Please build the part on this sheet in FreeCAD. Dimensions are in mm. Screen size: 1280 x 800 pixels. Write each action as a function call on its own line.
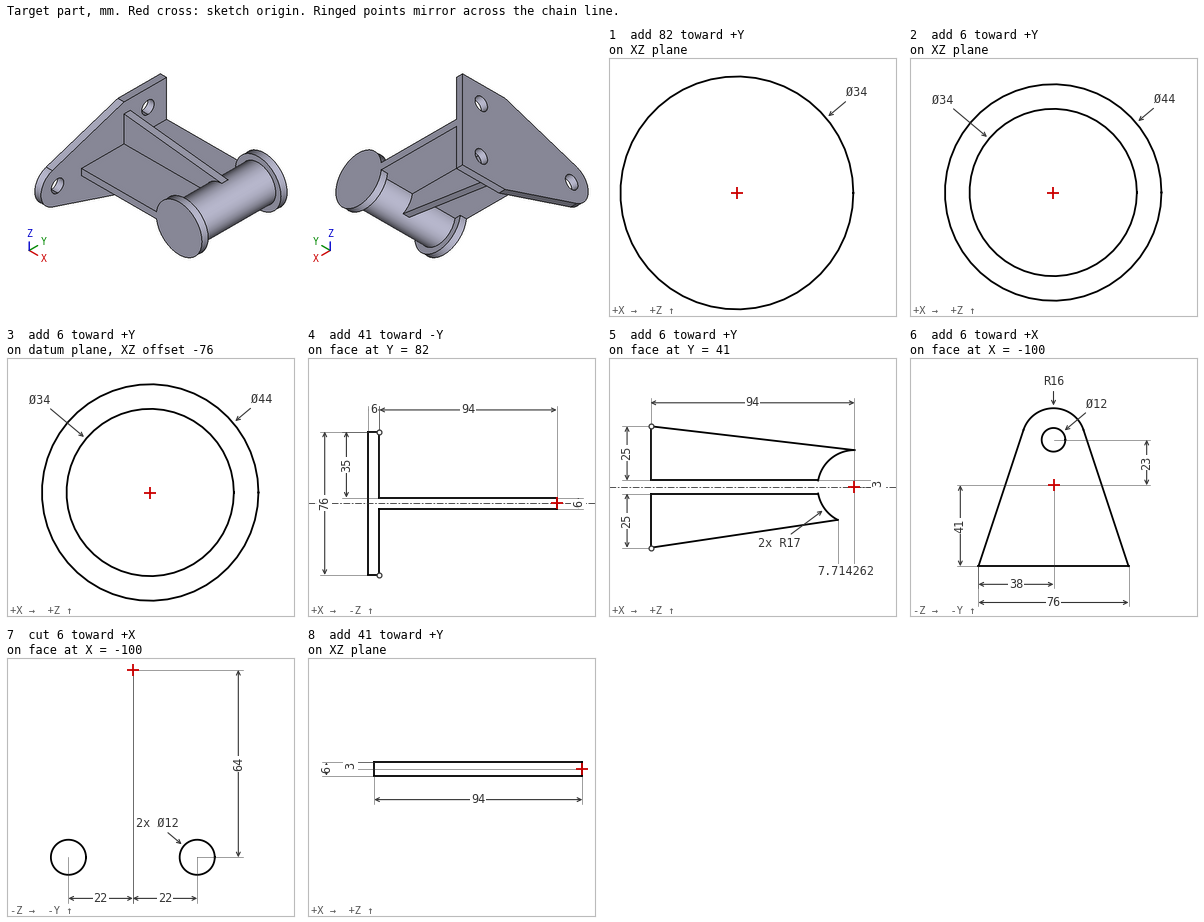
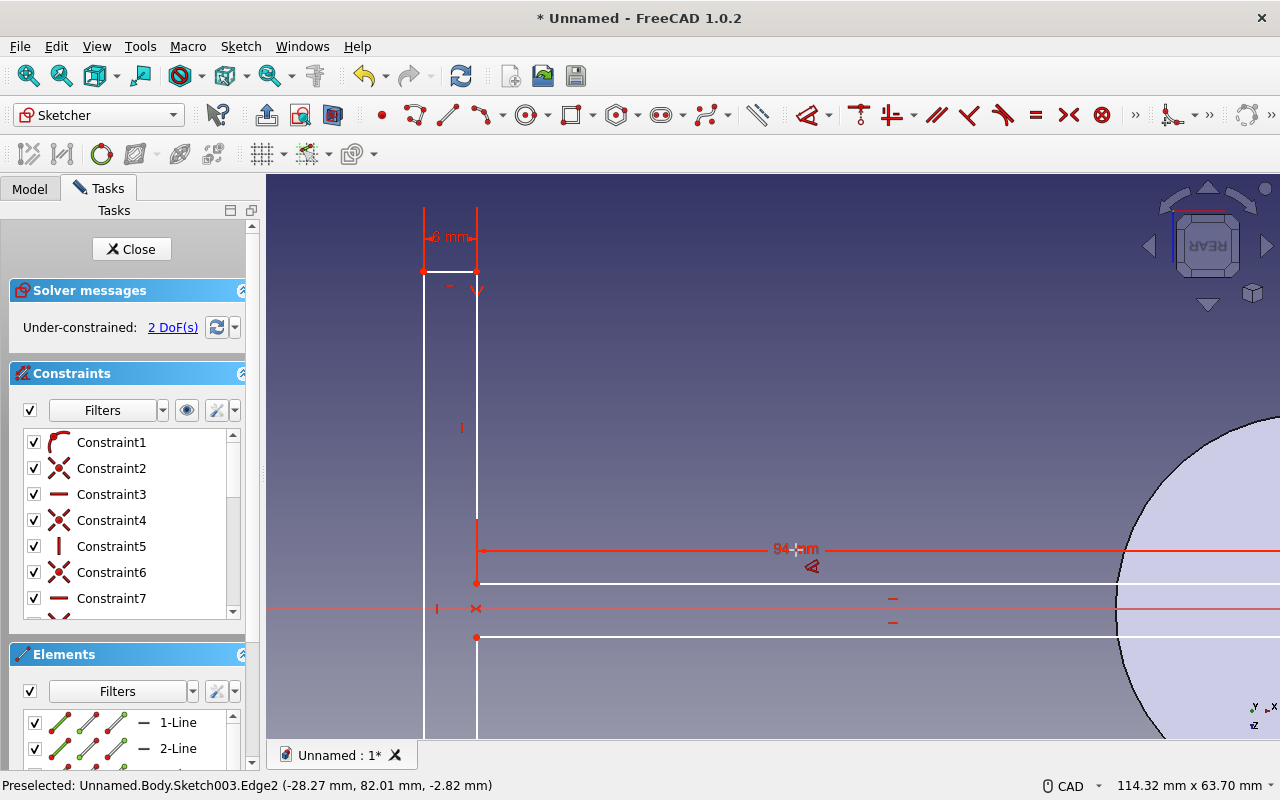
click(477, 490)
click(443, 428)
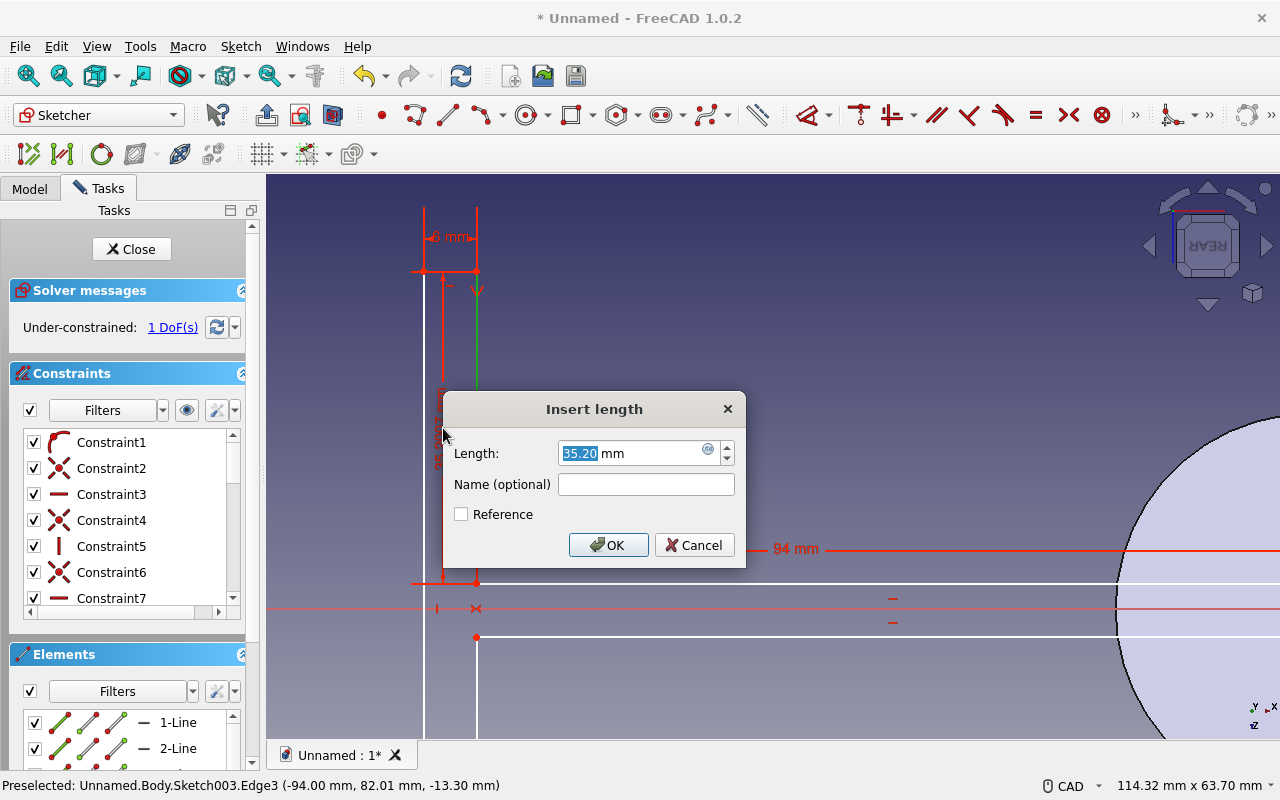
text(35)
key(Return)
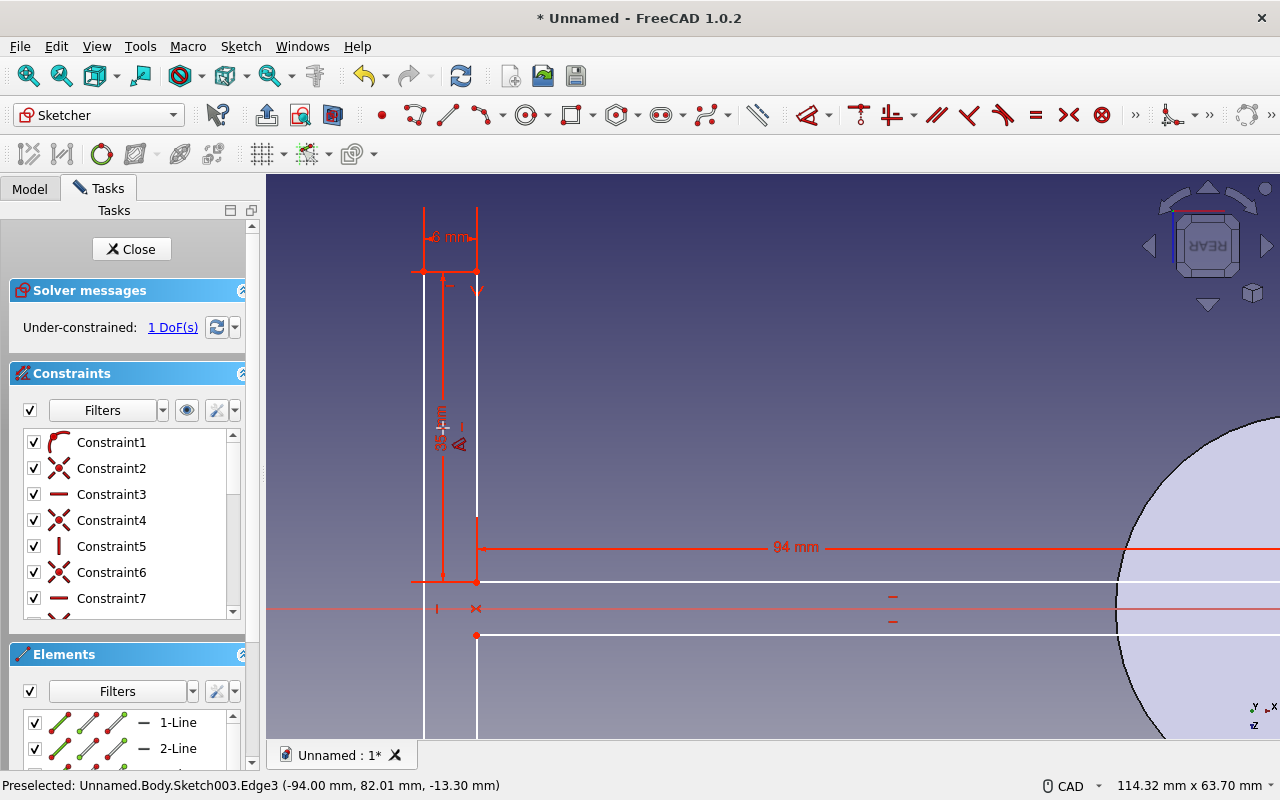
click(424, 474)
click(390, 491)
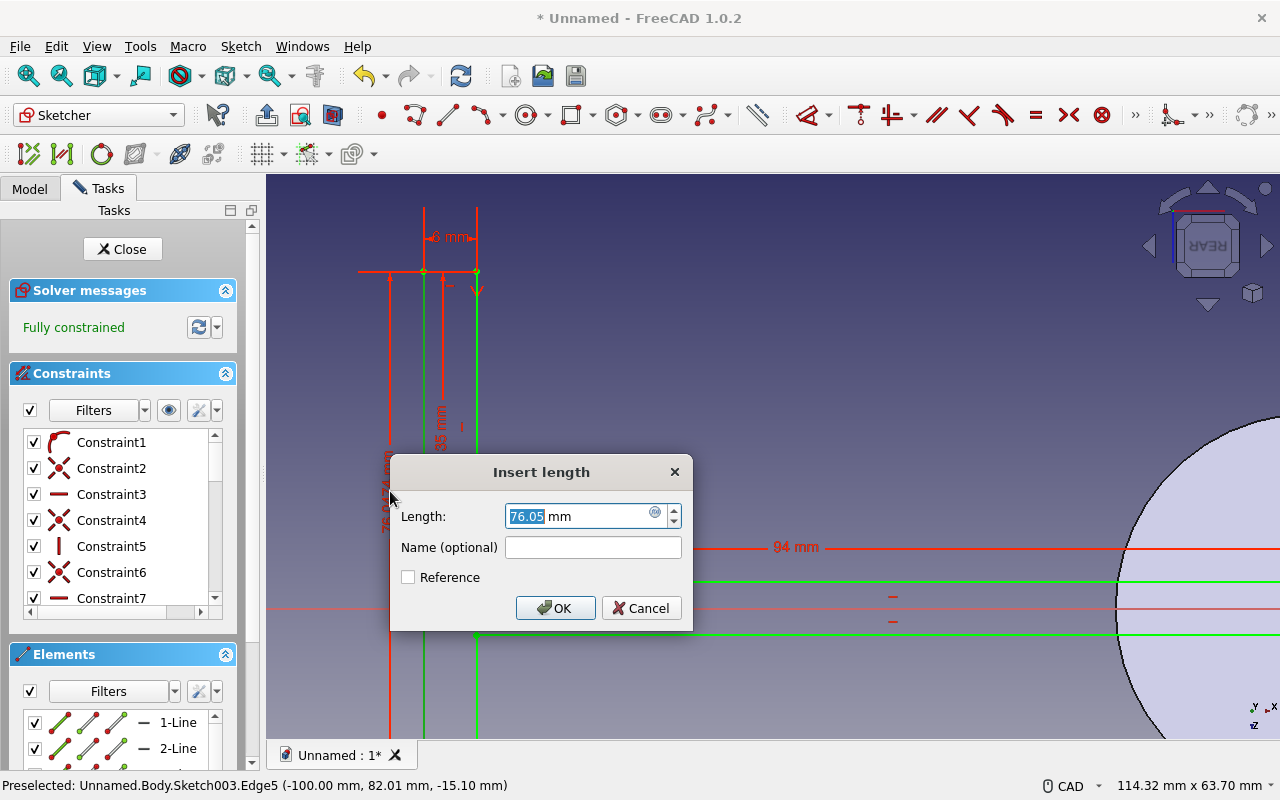
text(76)
key(Return)
key(Escape)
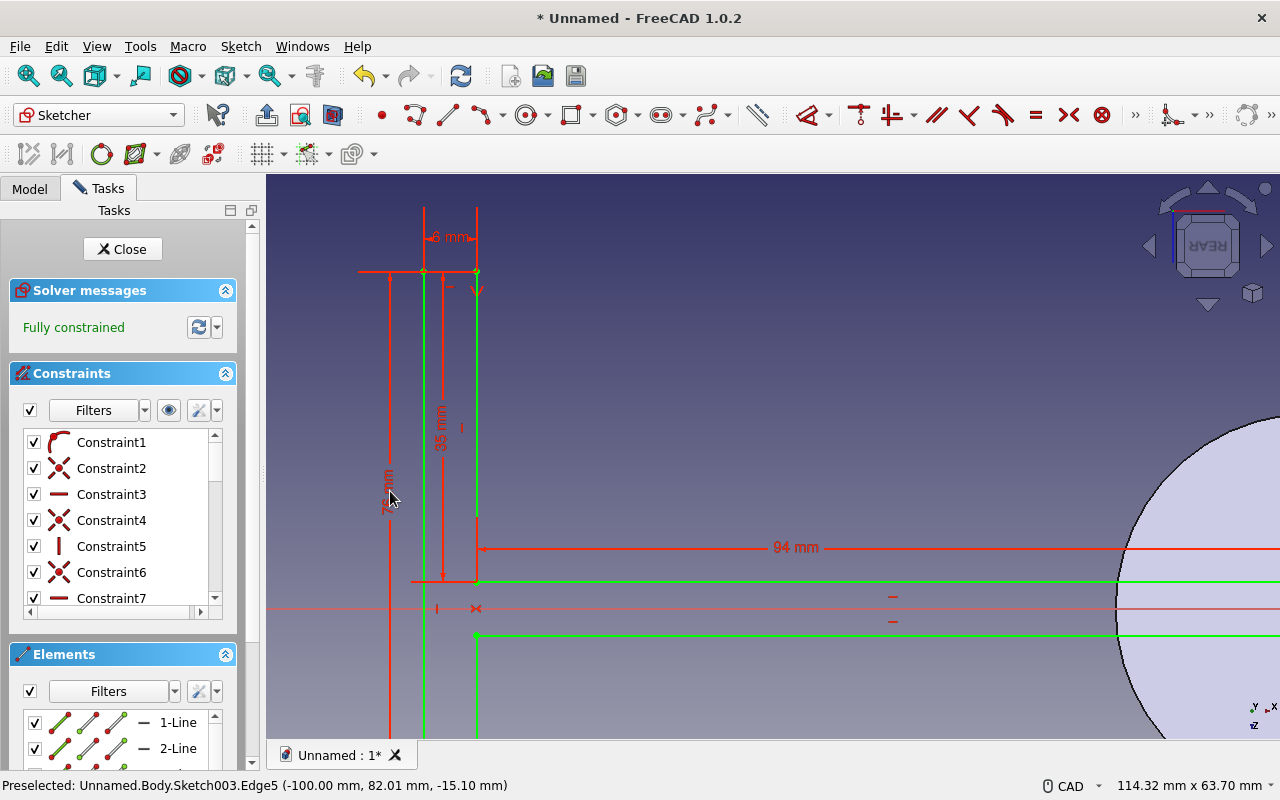
click(123, 249)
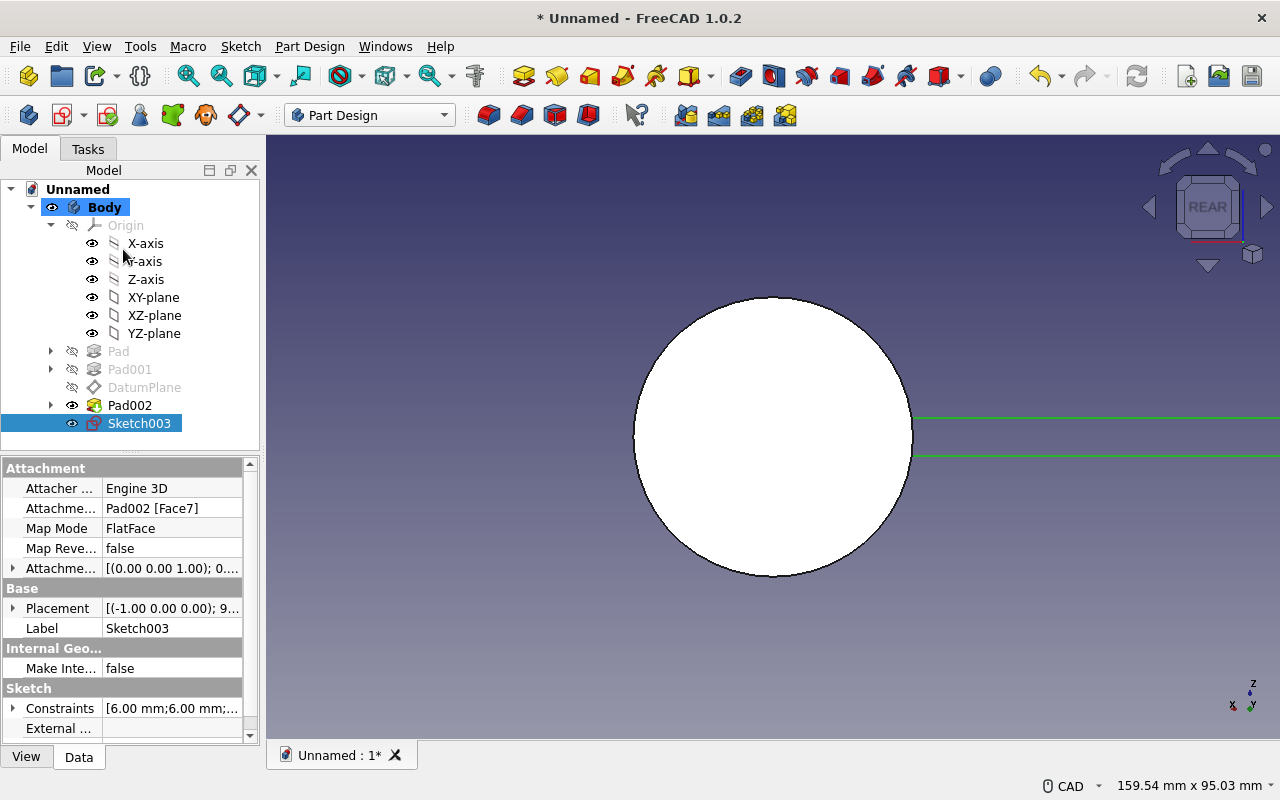
click(524, 76)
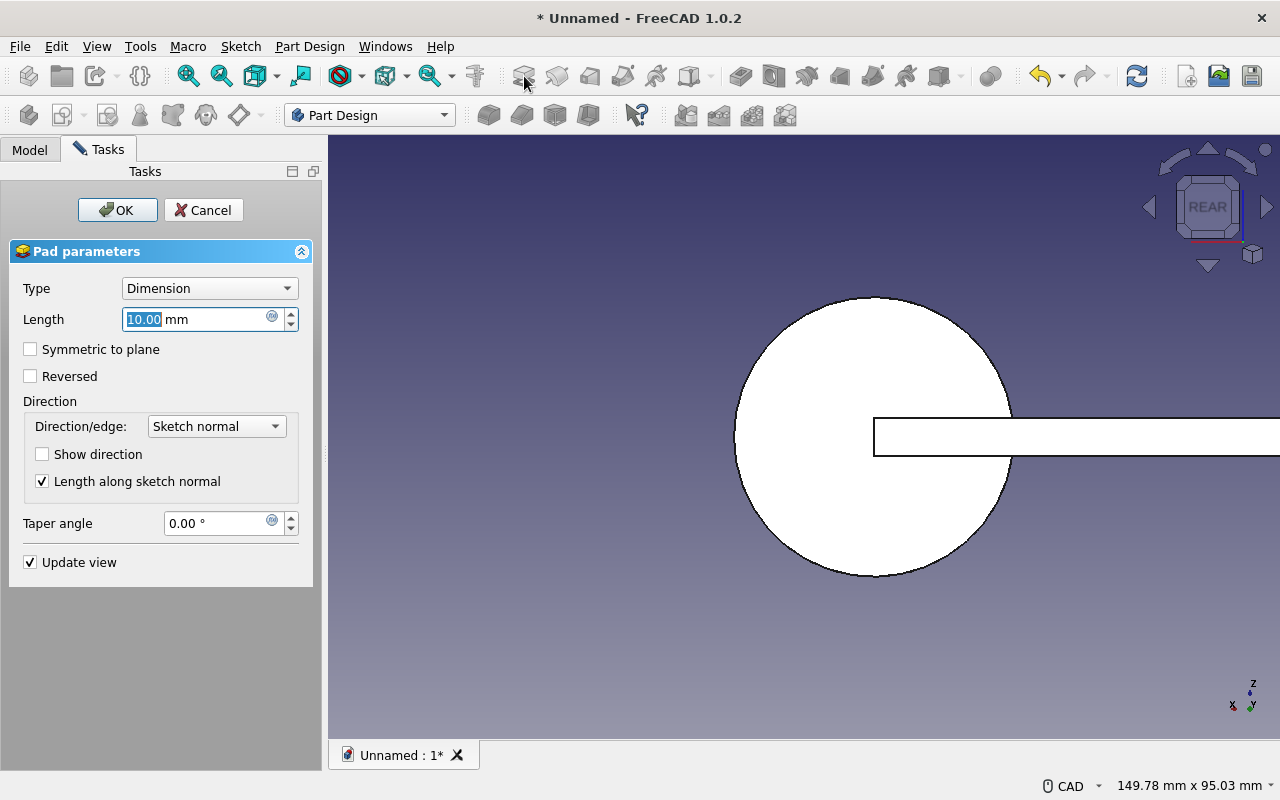
text(41)
key(Tab)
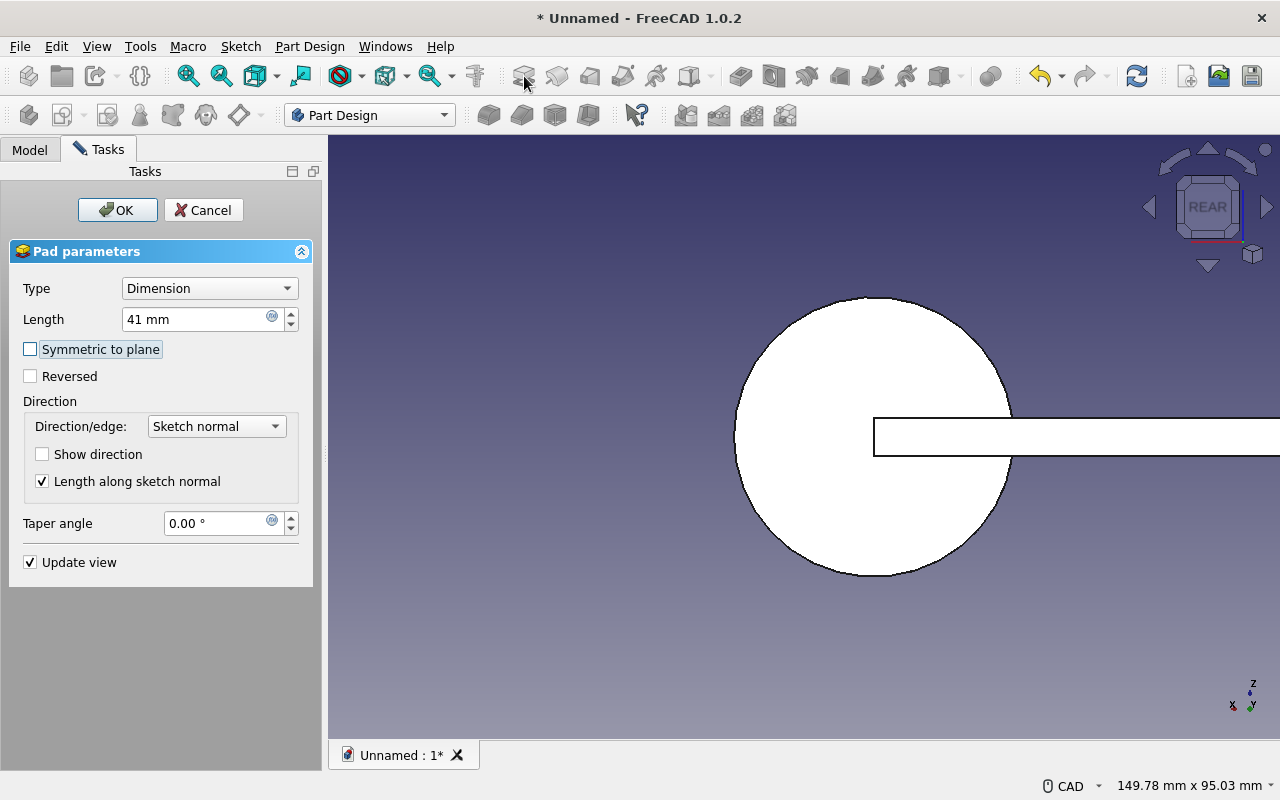
click(31, 376)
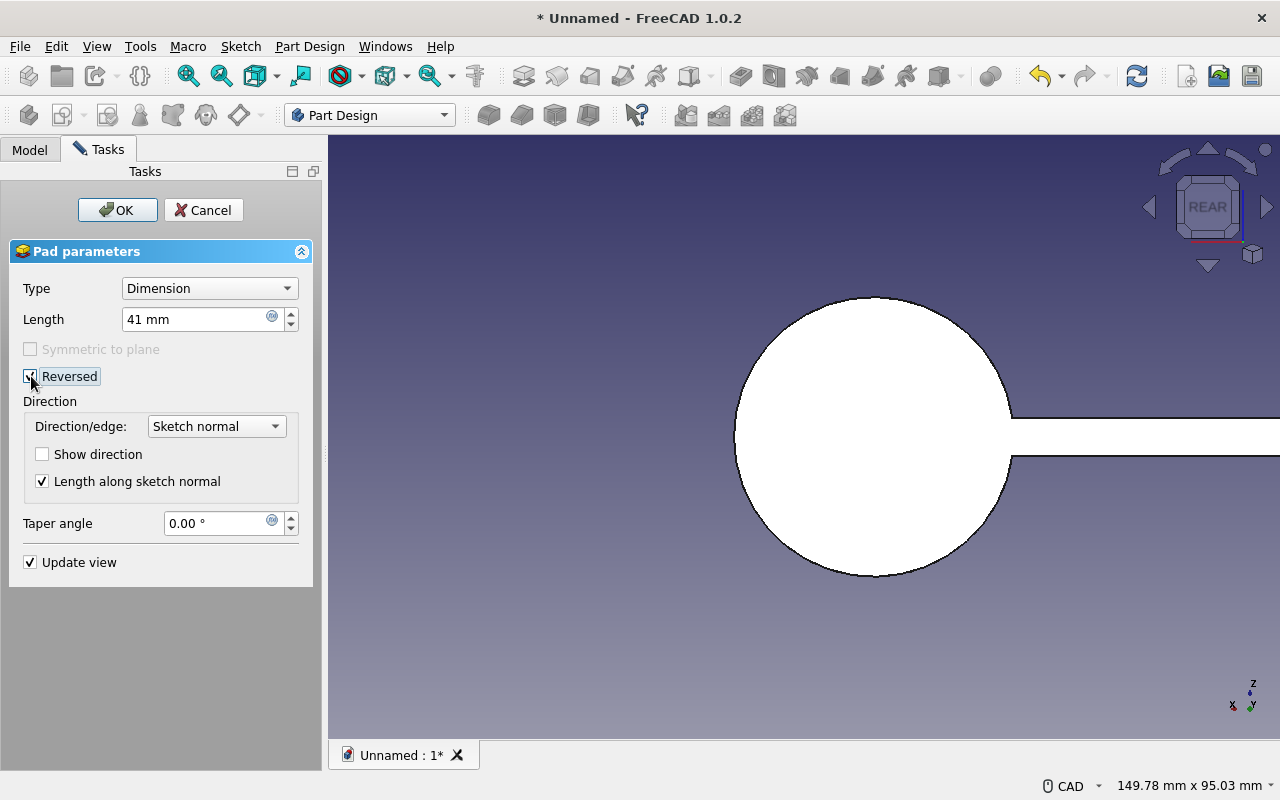
click(118, 210)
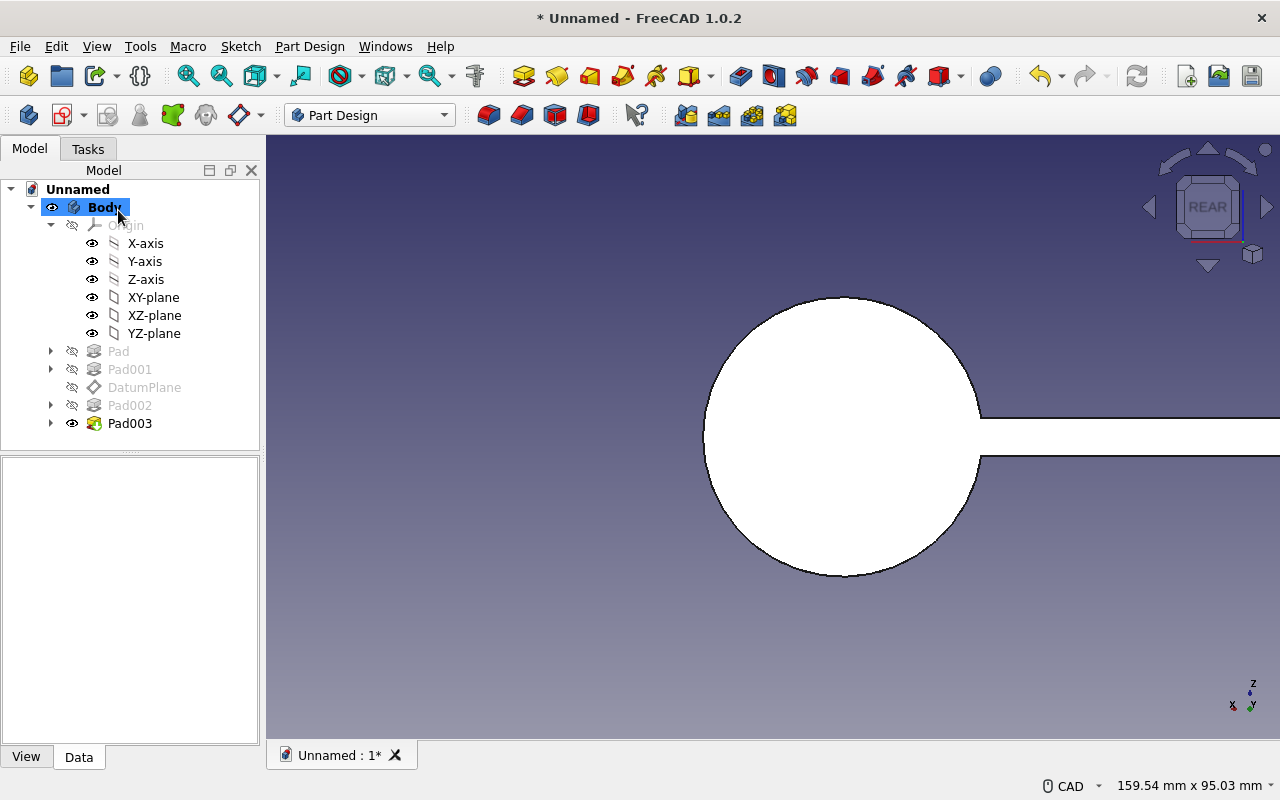
click(189, 76)